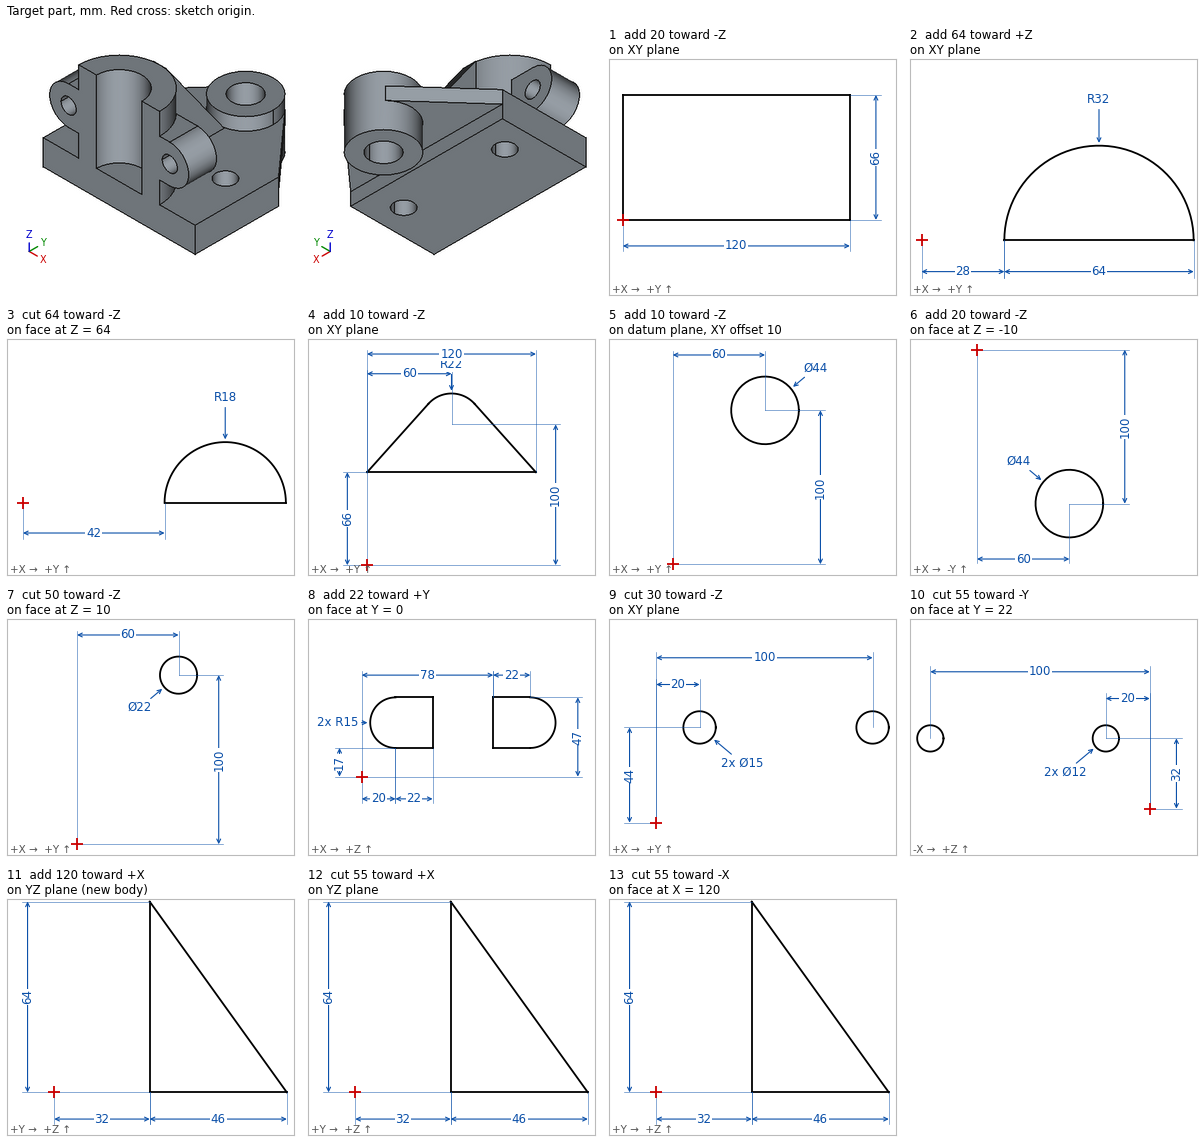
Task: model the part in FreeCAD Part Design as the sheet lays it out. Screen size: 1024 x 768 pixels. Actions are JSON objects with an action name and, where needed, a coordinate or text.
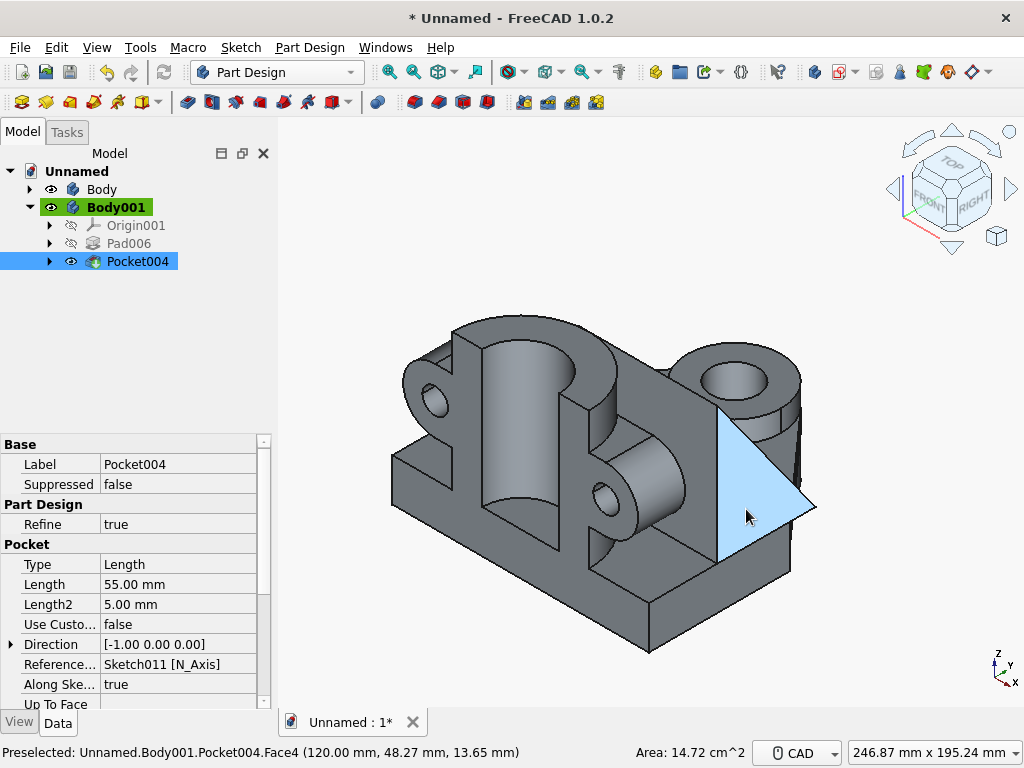
{"action": "left_click", "coordinate": [840, 72]}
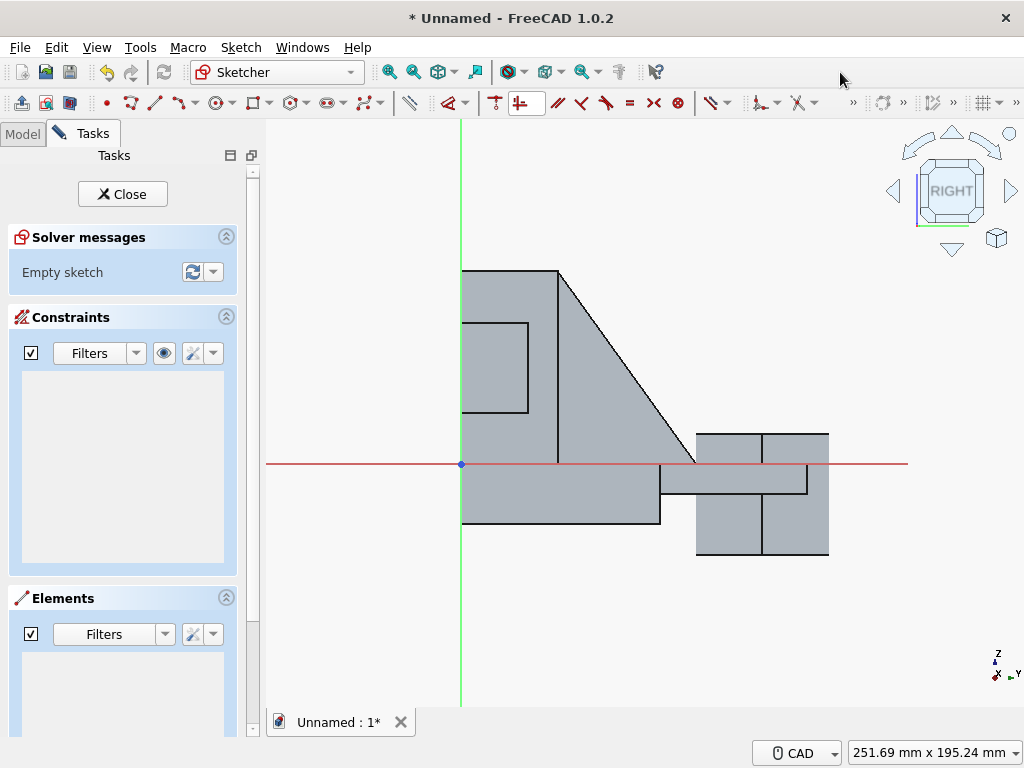
{"action": "scroll", "coordinate": [581, 313], "scroll_direction": "up", "scroll_amount": 3}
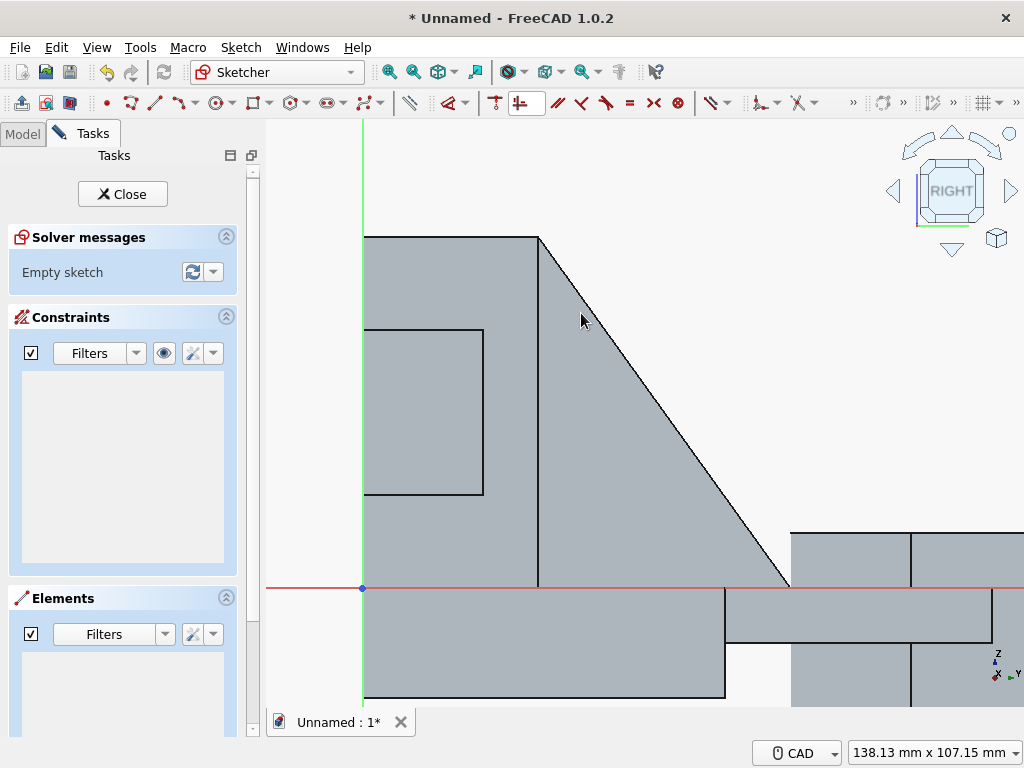
{"action": "left_click", "coordinate": [132, 104]}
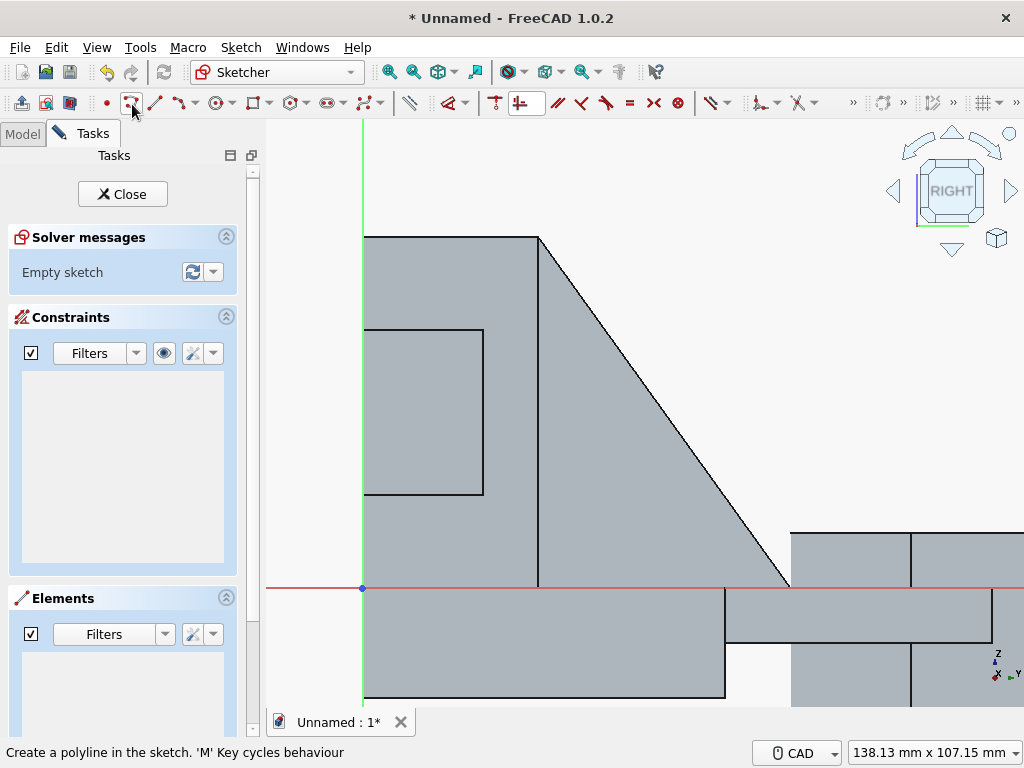
{"action": "left_click", "coordinate": [538, 588]}
{"action": "left_click", "coordinate": [791, 579]}
{"action": "left_click", "coordinate": [538, 237]}
{"action": "left_click", "coordinate": [538, 588]}
{"action": "key", "text": "Escape"}
{"action": "key", "text": "Escape"}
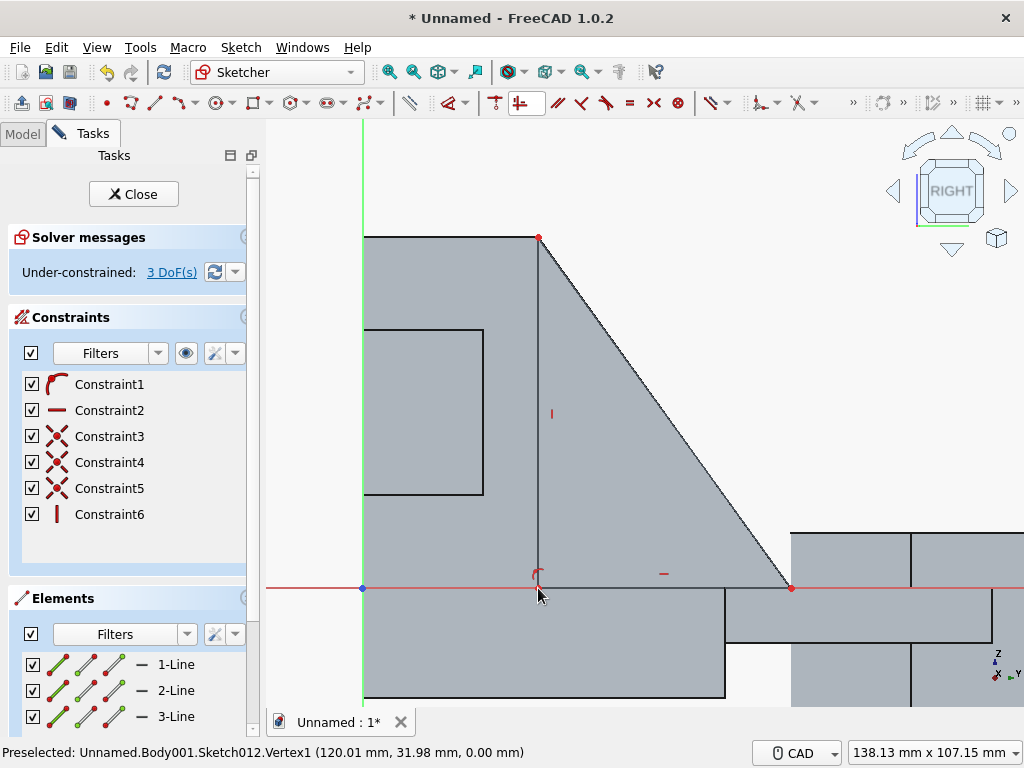
{"action": "left_click", "coordinate": [448, 104]}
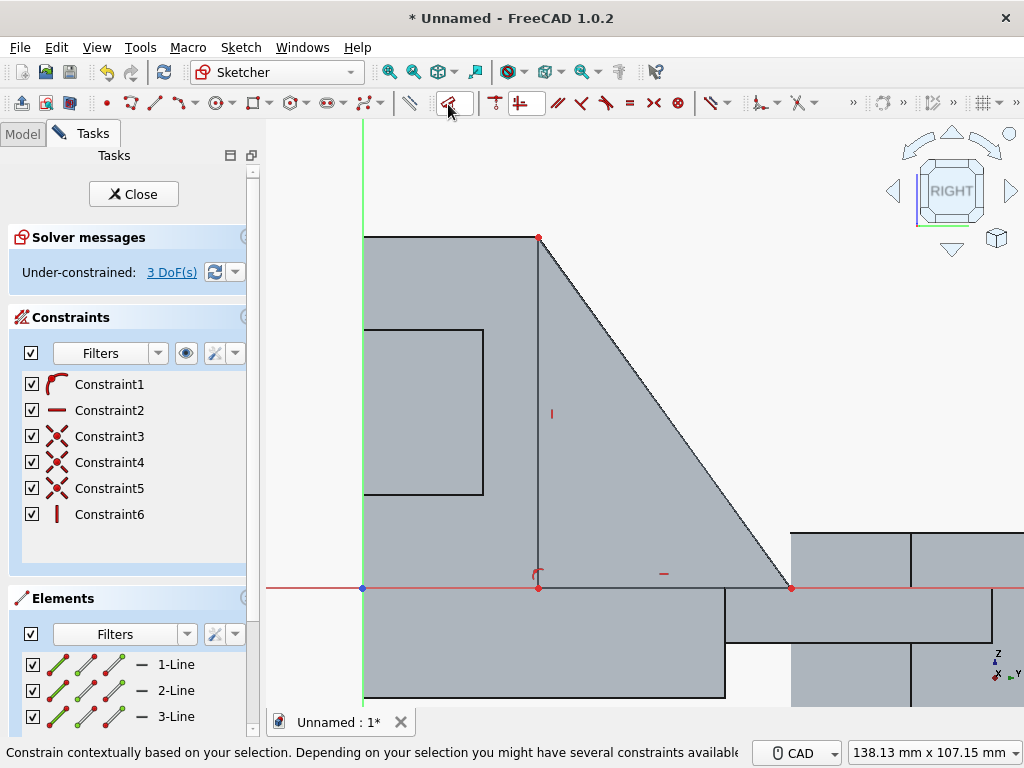
{"action": "left_click", "coordinate": [614, 588]}
{"action": "left_click", "coordinate": [664, 622]}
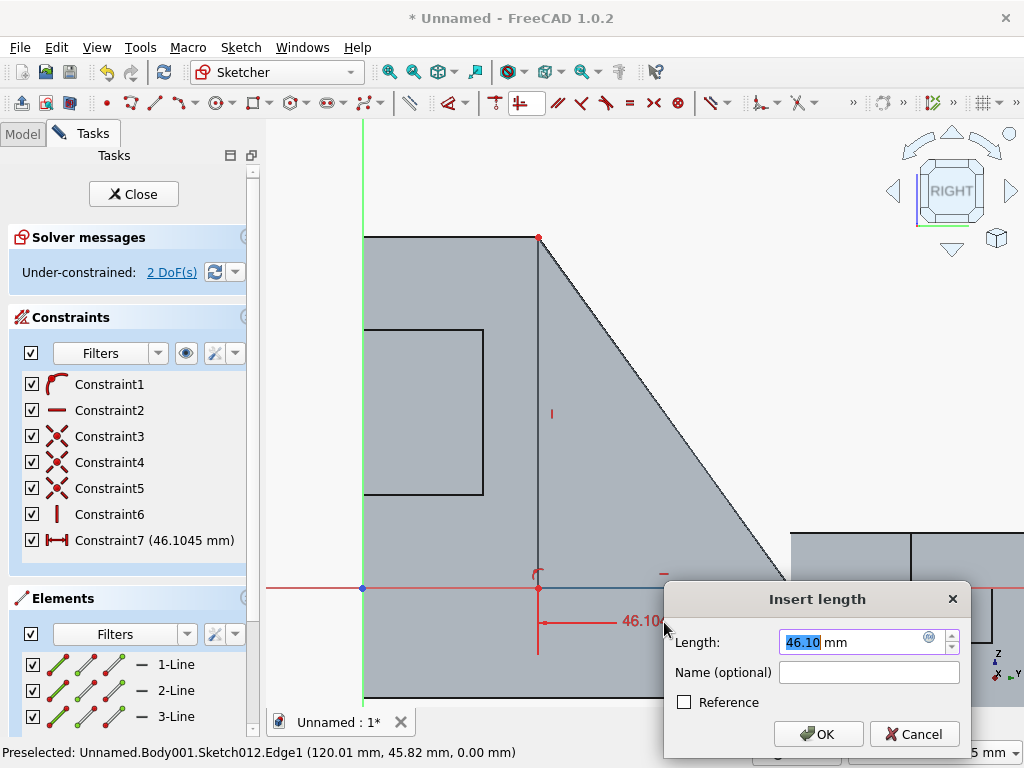
{"action": "type", "text": "46"}
{"action": "key", "text": "Return"}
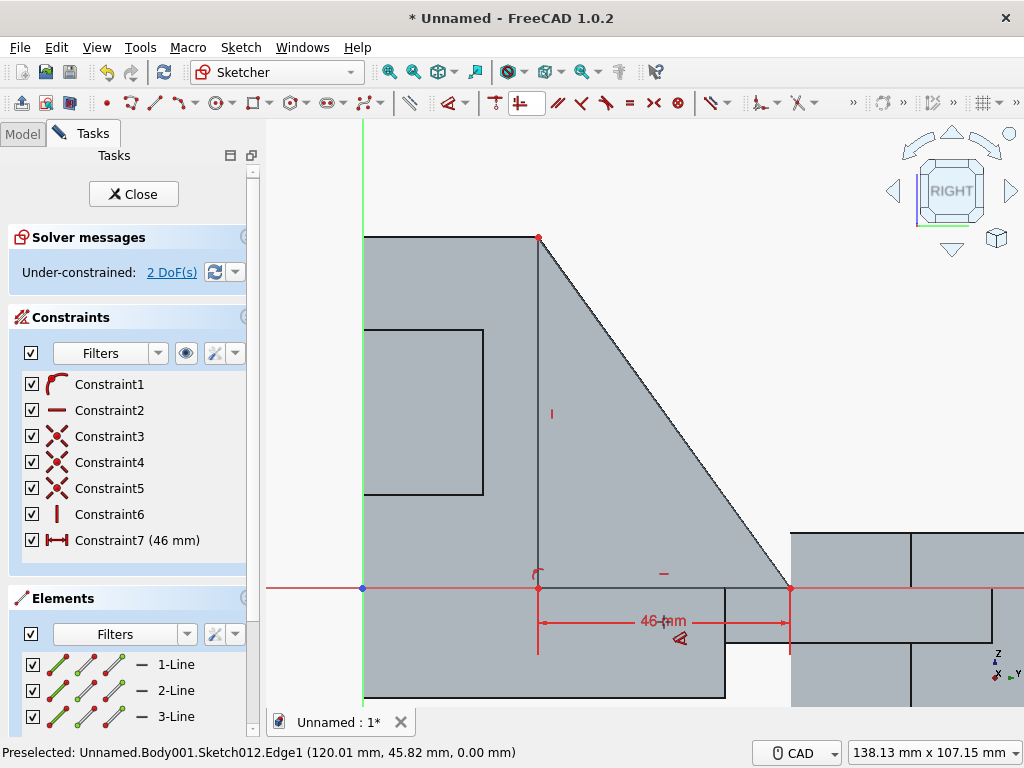
{"action": "left_click", "coordinate": [538, 343]}
{"action": "left_click", "coordinate": [504, 413]}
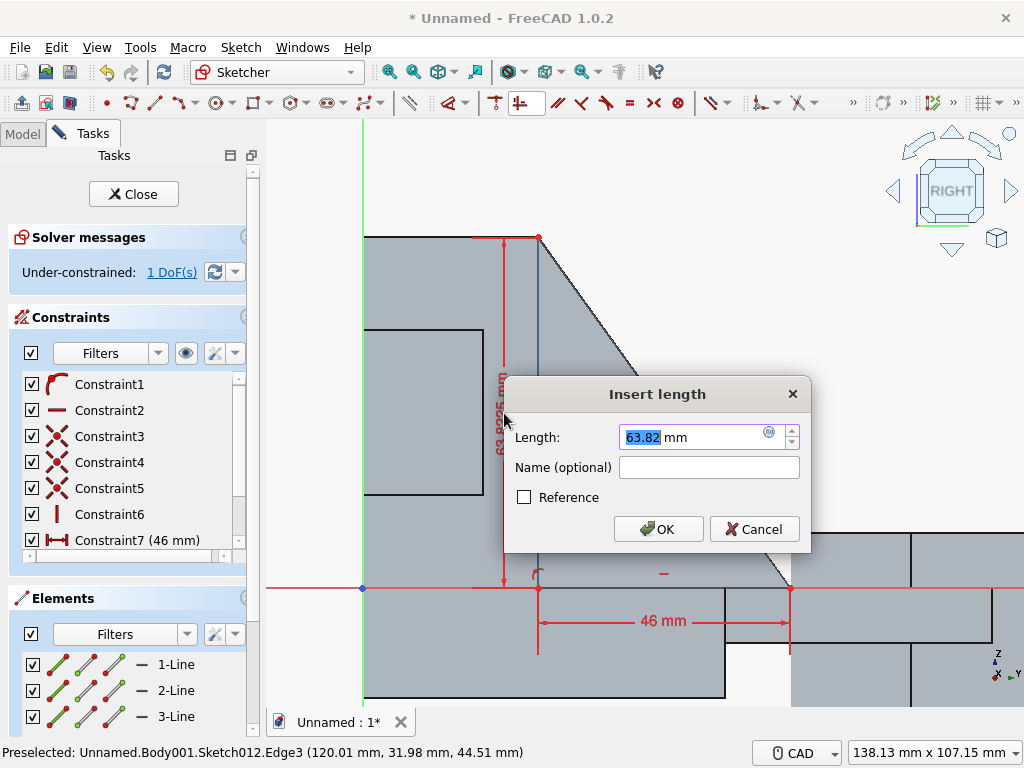
{"action": "type", "text": "64"}
{"action": "key", "text": "Return"}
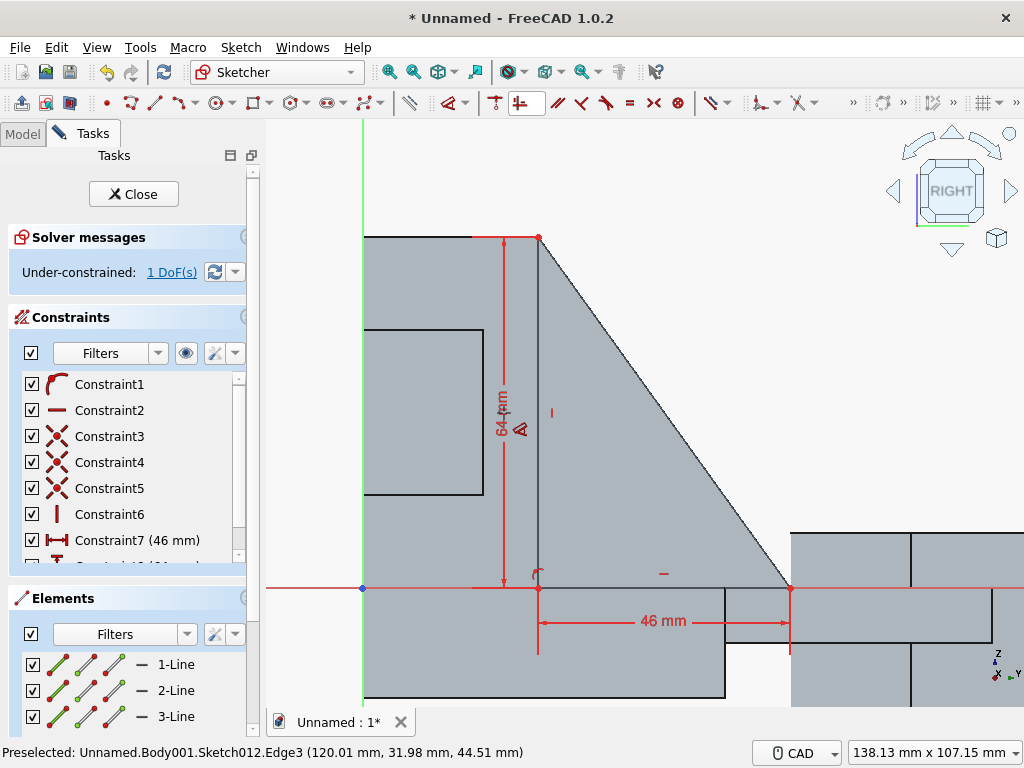
{"action": "left_click", "coordinate": [538, 588]}
{"action": "left_click", "coordinate": [450, 622]}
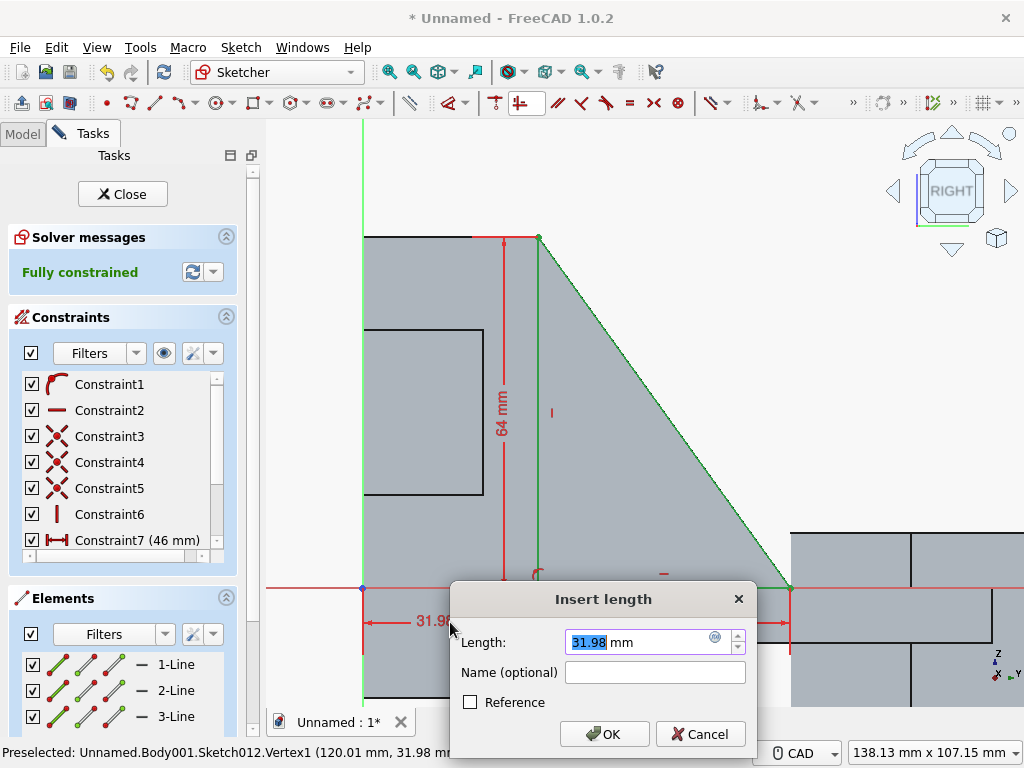
{"action": "type", "text": "32"}
{"action": "key", "text": "Return"}
{"action": "key", "text": "Escape"}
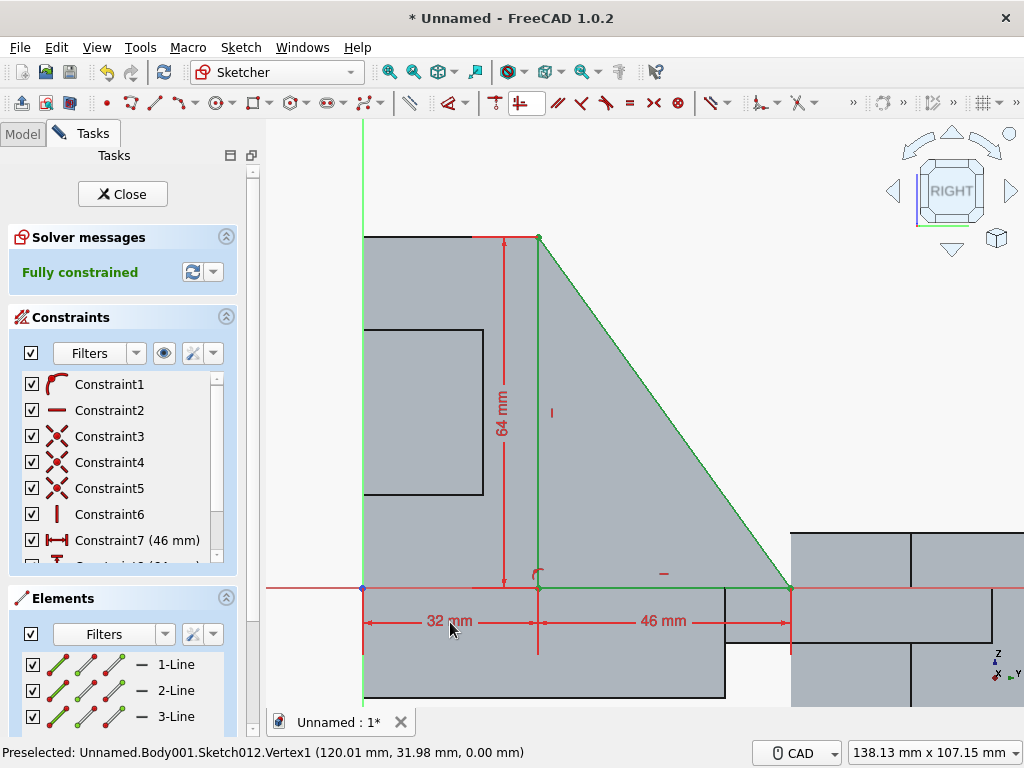
{"action": "left_click", "coordinate": [123, 194]}